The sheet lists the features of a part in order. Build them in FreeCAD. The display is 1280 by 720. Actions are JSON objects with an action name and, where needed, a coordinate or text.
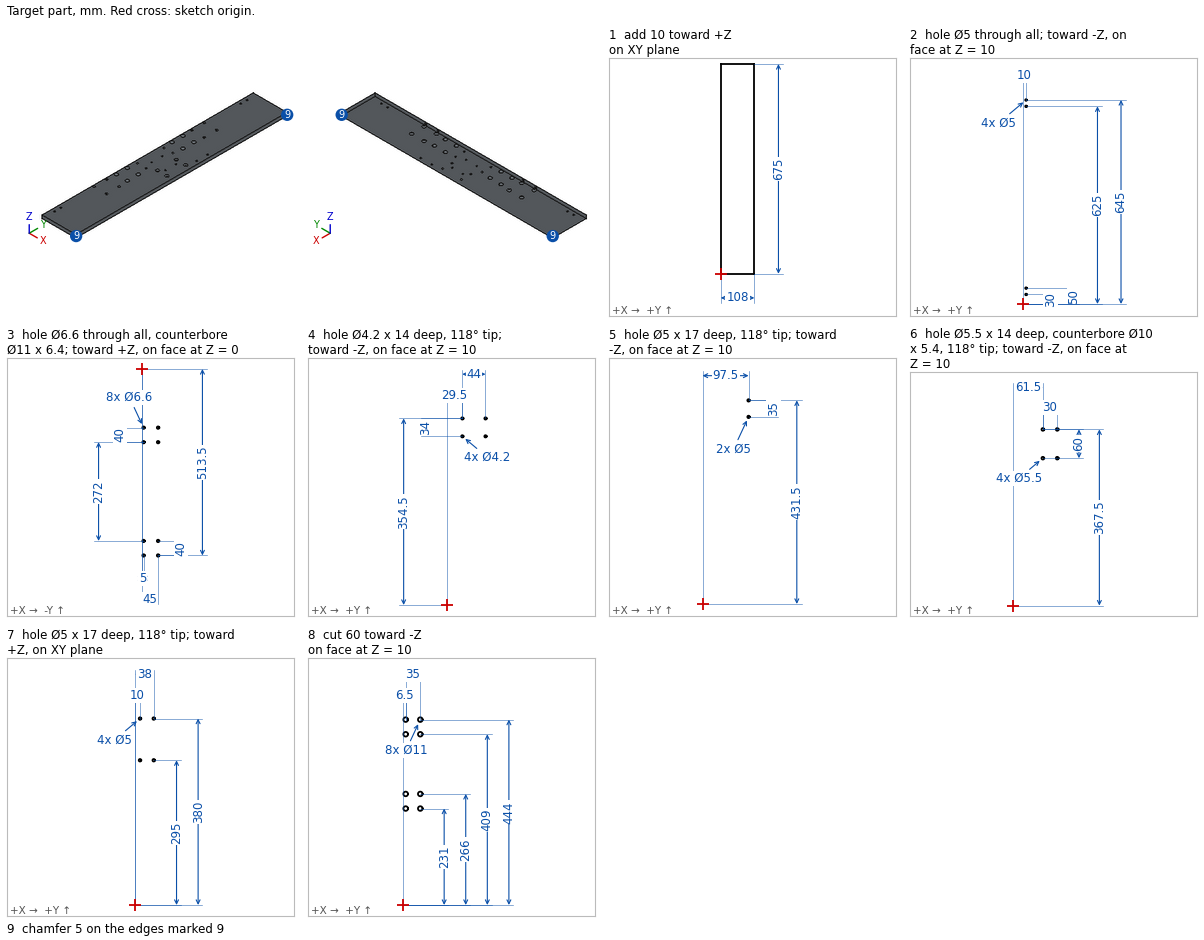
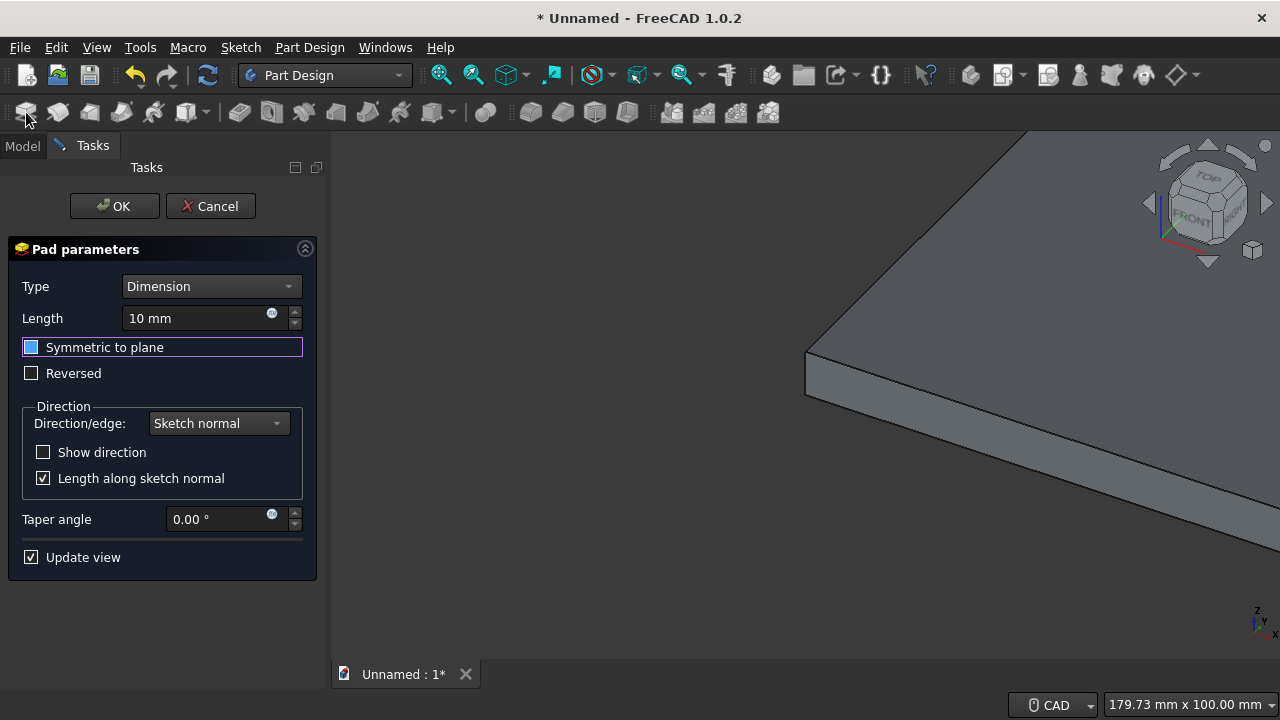
{"action": "left_click", "coordinate": [115, 206]}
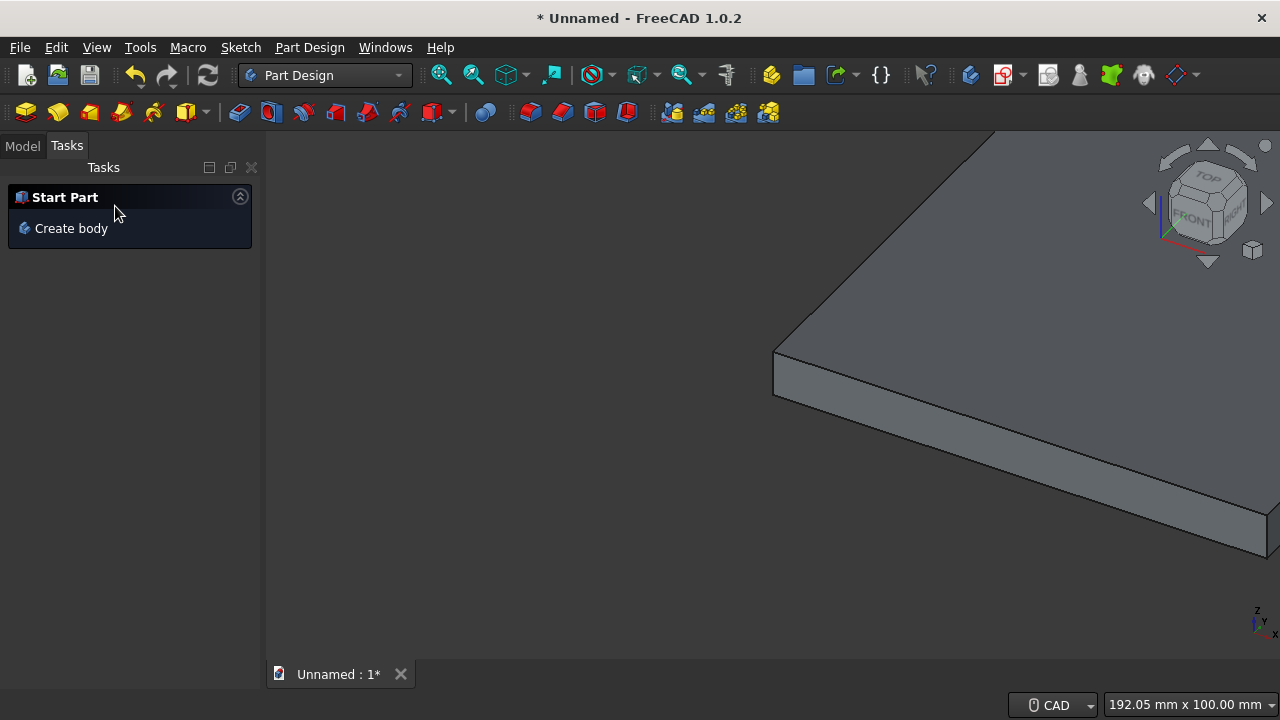
{"action": "left_click", "coordinate": [442, 76]}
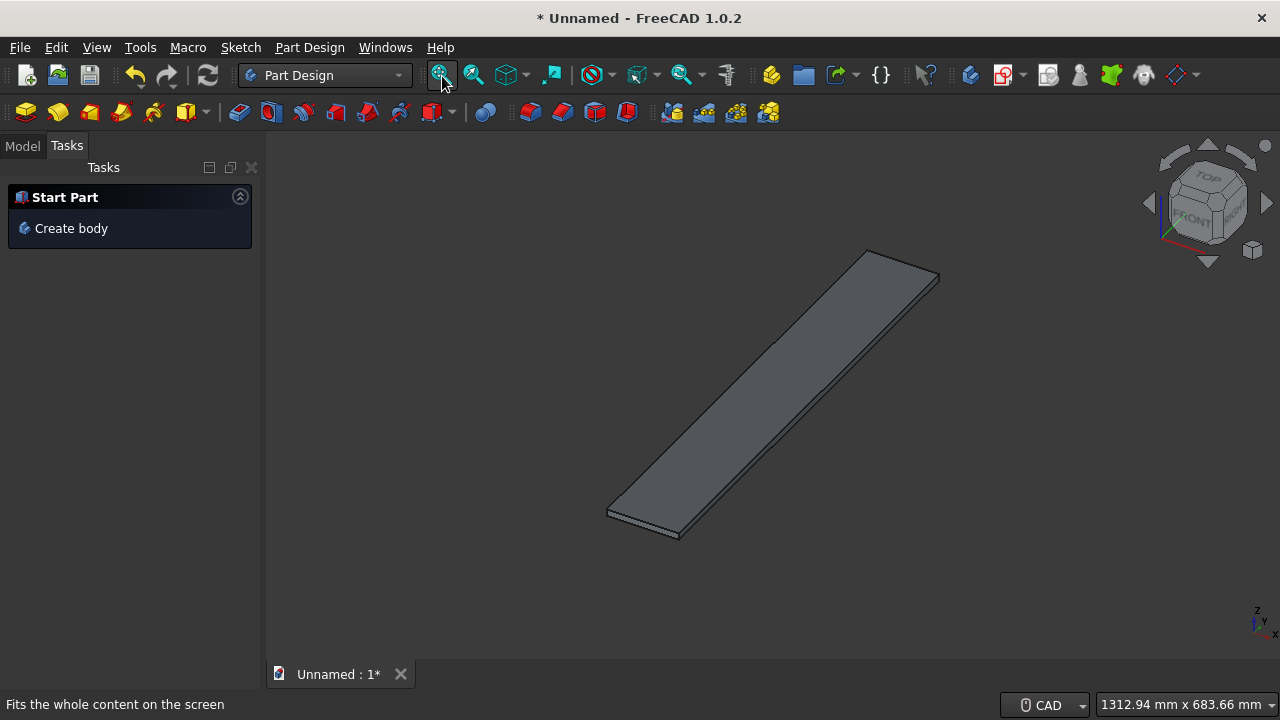
{"action": "left_click", "coordinate": [847, 317]}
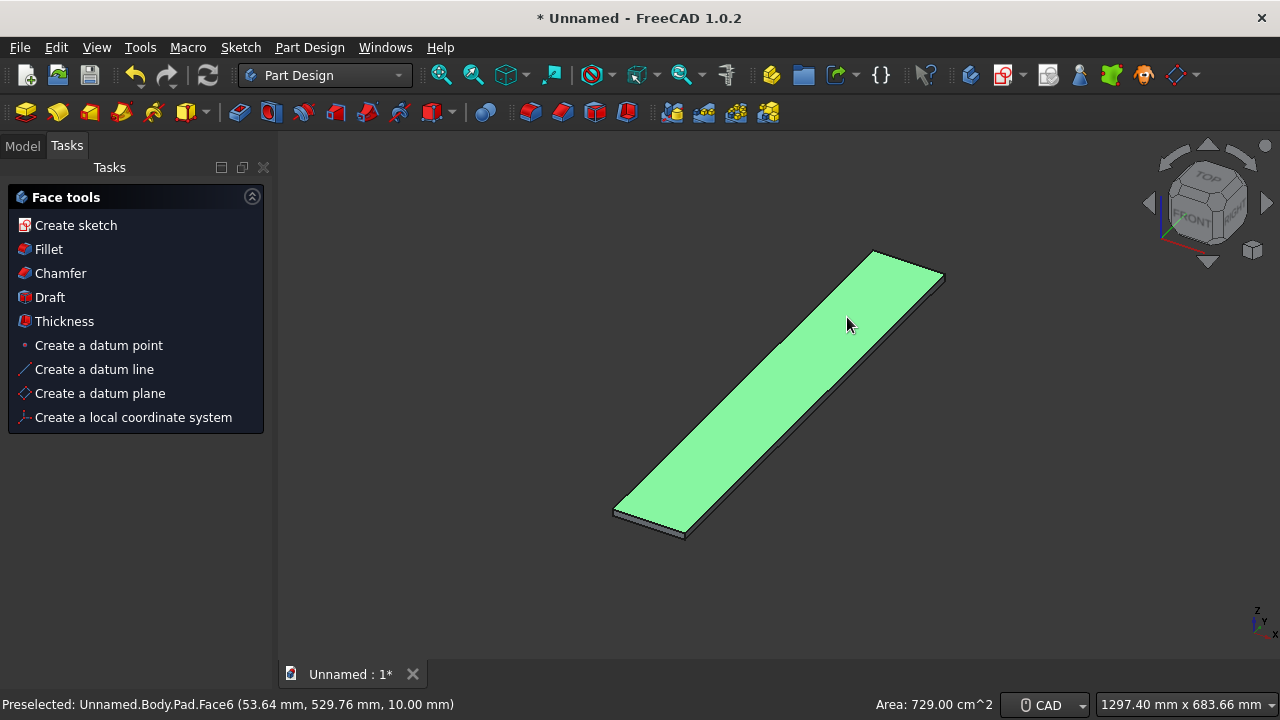
{"action": "left_click", "coordinate": [1004, 76]}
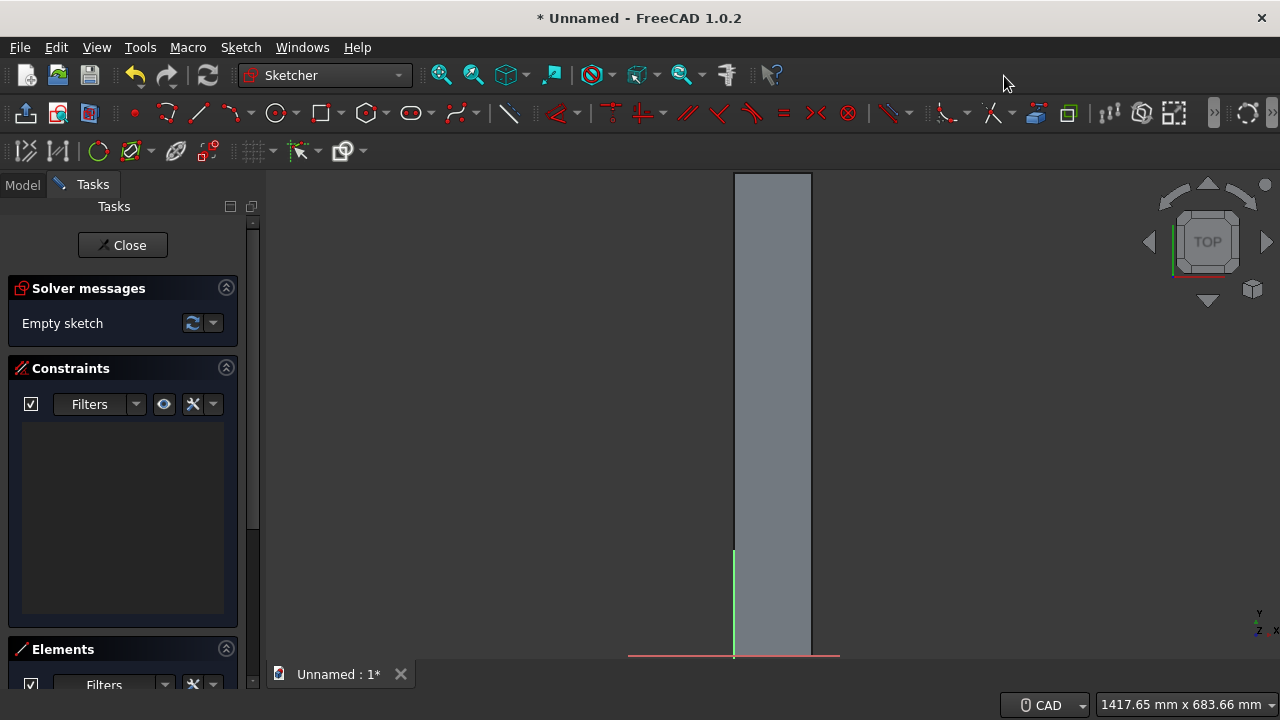
{"action": "scroll", "coordinate": [635, 395], "scroll_direction": "down", "scroll_amount": 2}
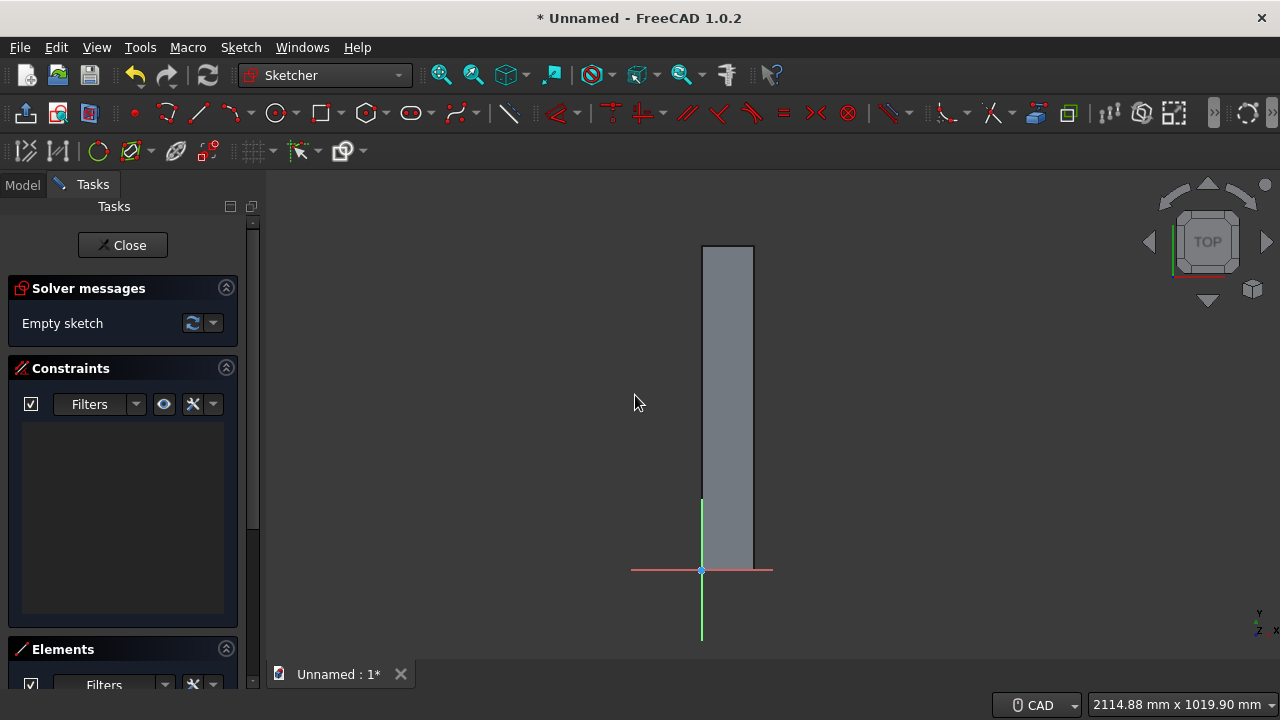
{"action": "left_click", "coordinate": [276, 114]}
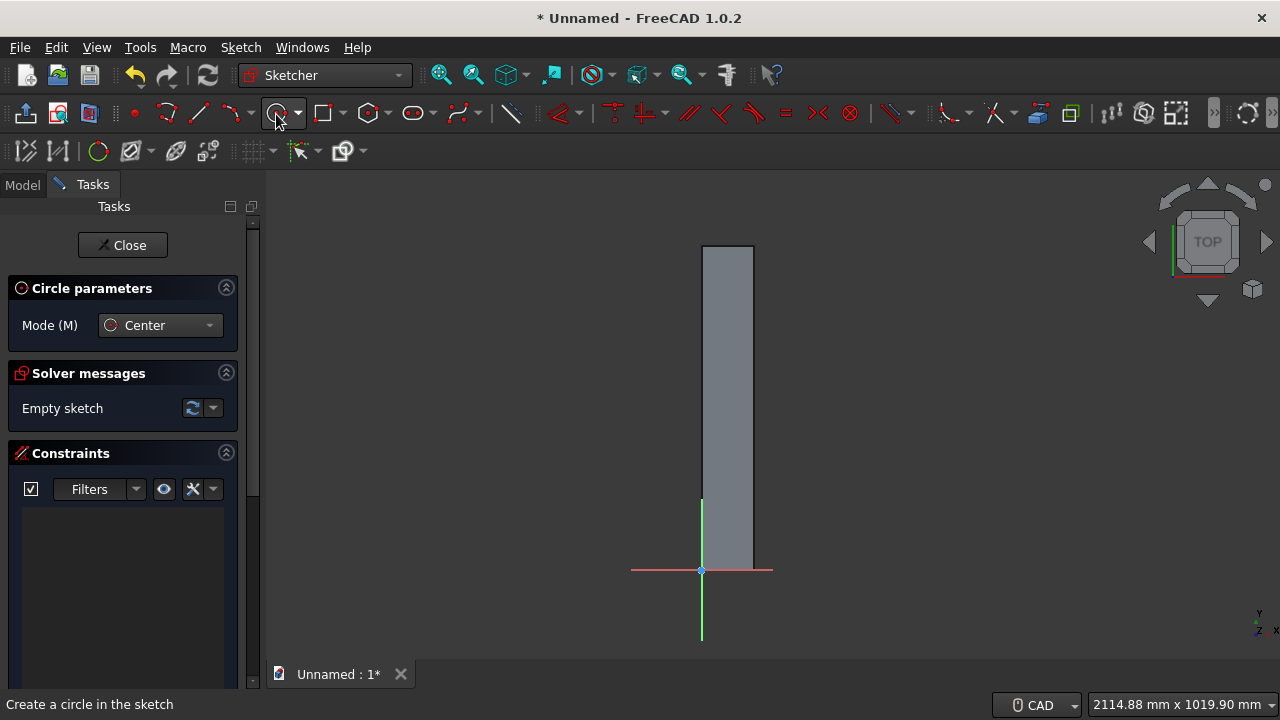
{"action": "scroll", "coordinate": [707, 261], "scroll_direction": "up", "scroll_amount": 15}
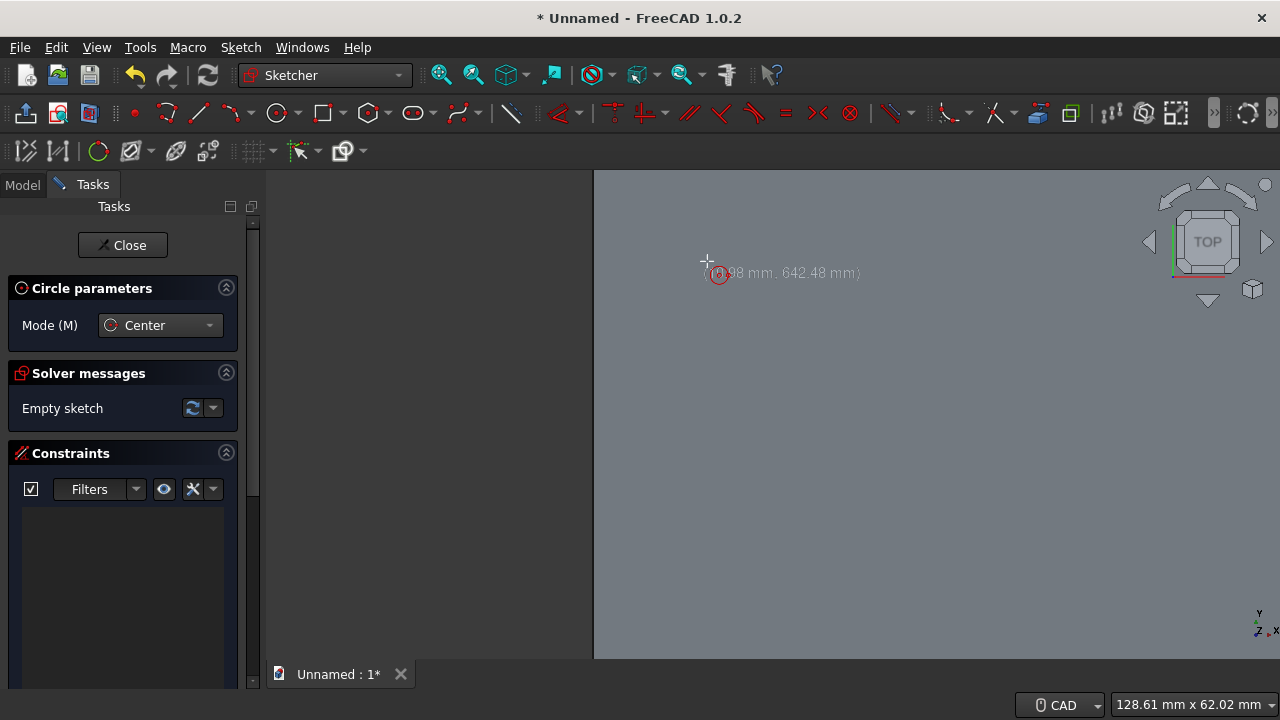
{"action": "scroll", "coordinate": [707, 261], "scroll_direction": "down", "scroll_amount": 15}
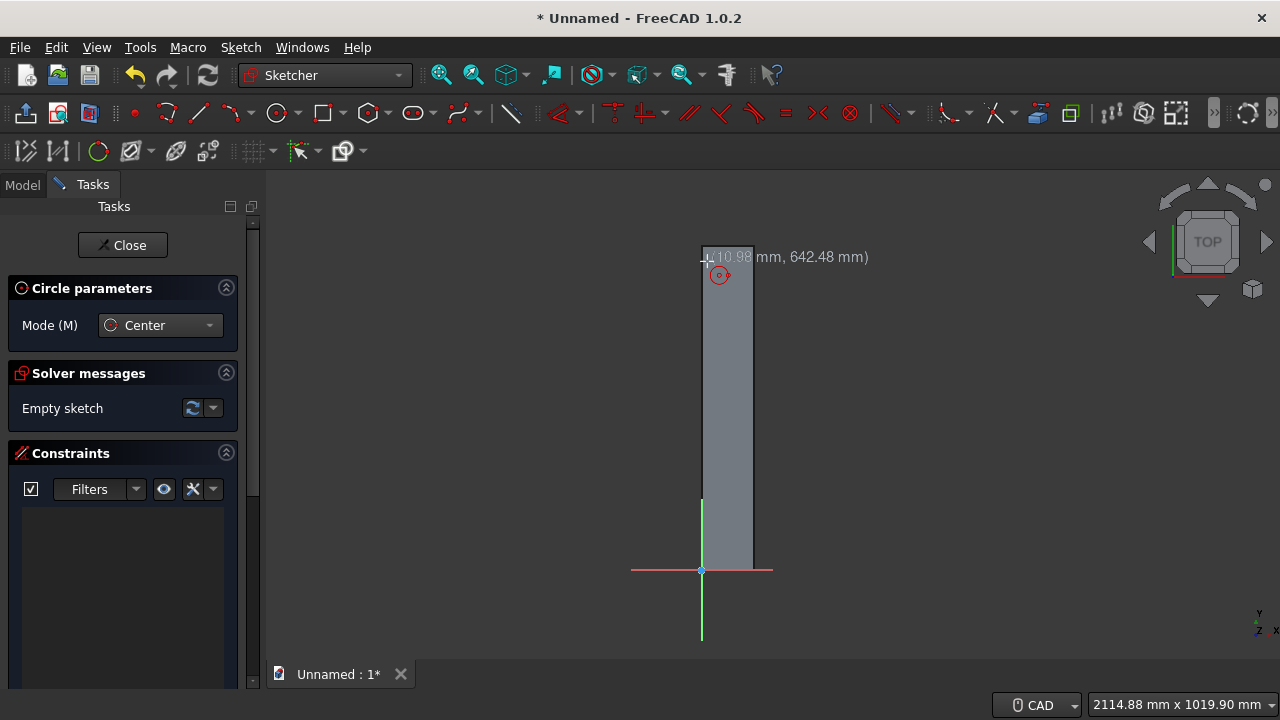
{"action": "scroll", "coordinate": [707, 261], "scroll_direction": "up", "scroll_amount": 6}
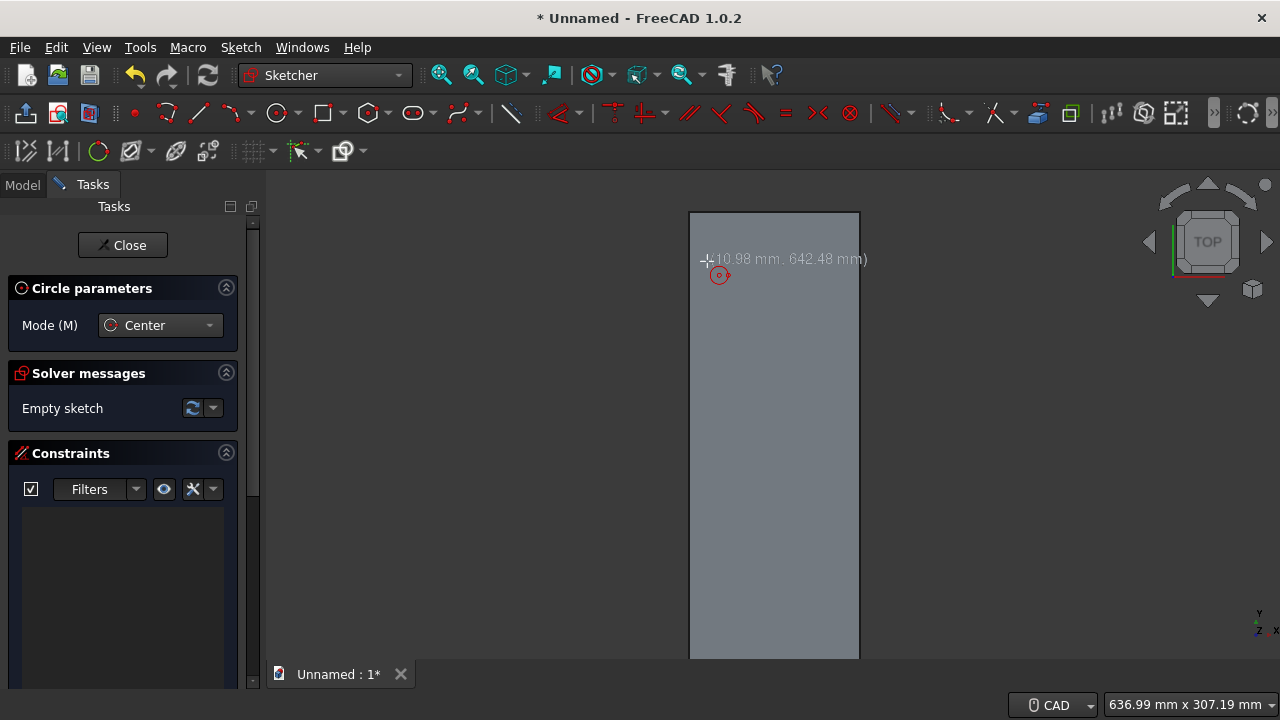
{"action": "left_click", "coordinate": [704, 260]}
{"action": "mouse_move", "coordinate": [707, 257]}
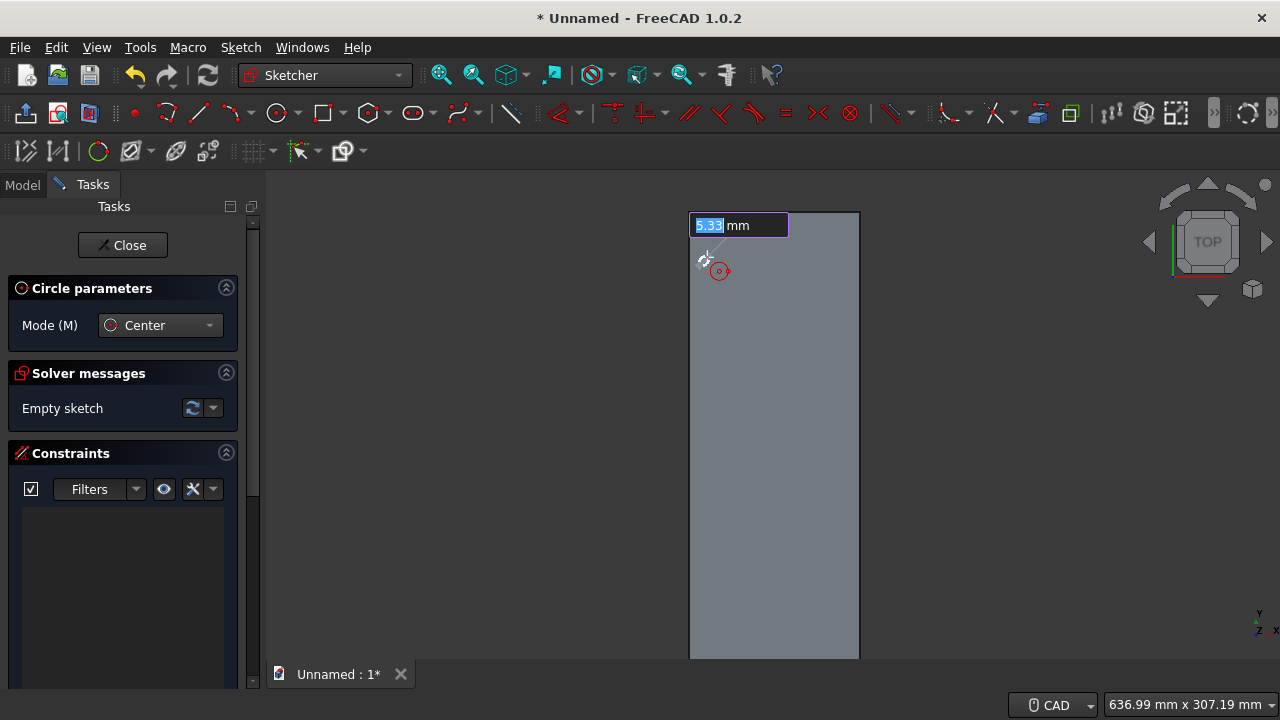
{"action": "type", "text": "5"}
{"action": "key", "text": "Return"}